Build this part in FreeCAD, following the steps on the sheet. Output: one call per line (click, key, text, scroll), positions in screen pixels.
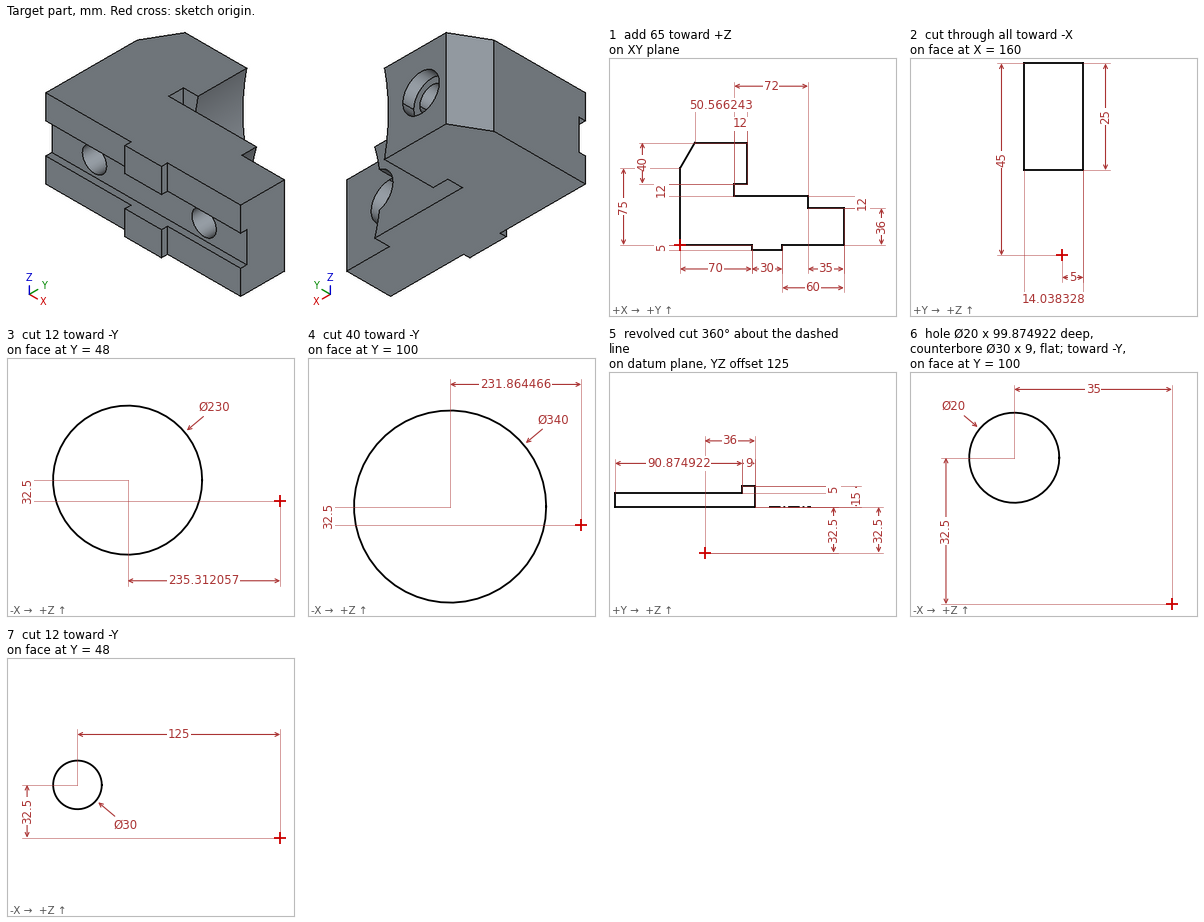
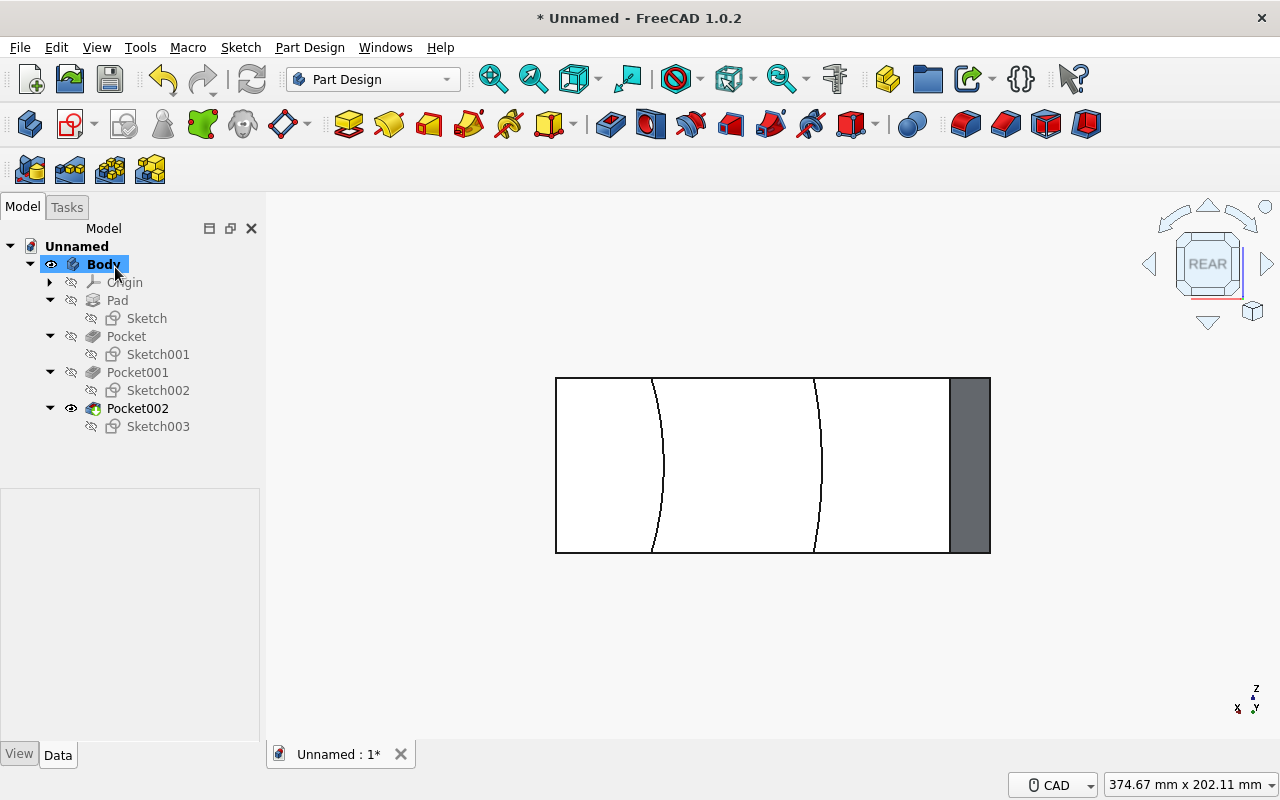
key(v)
key(f)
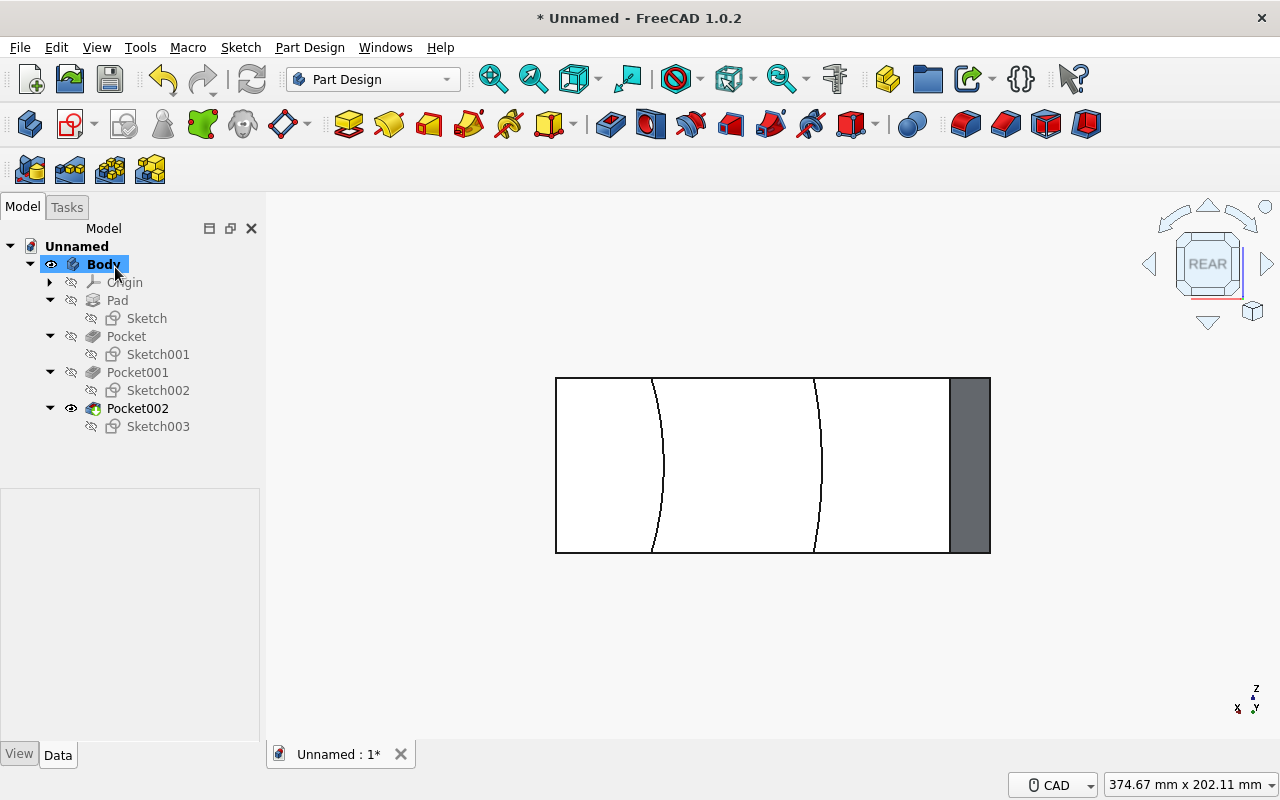
click(50, 282)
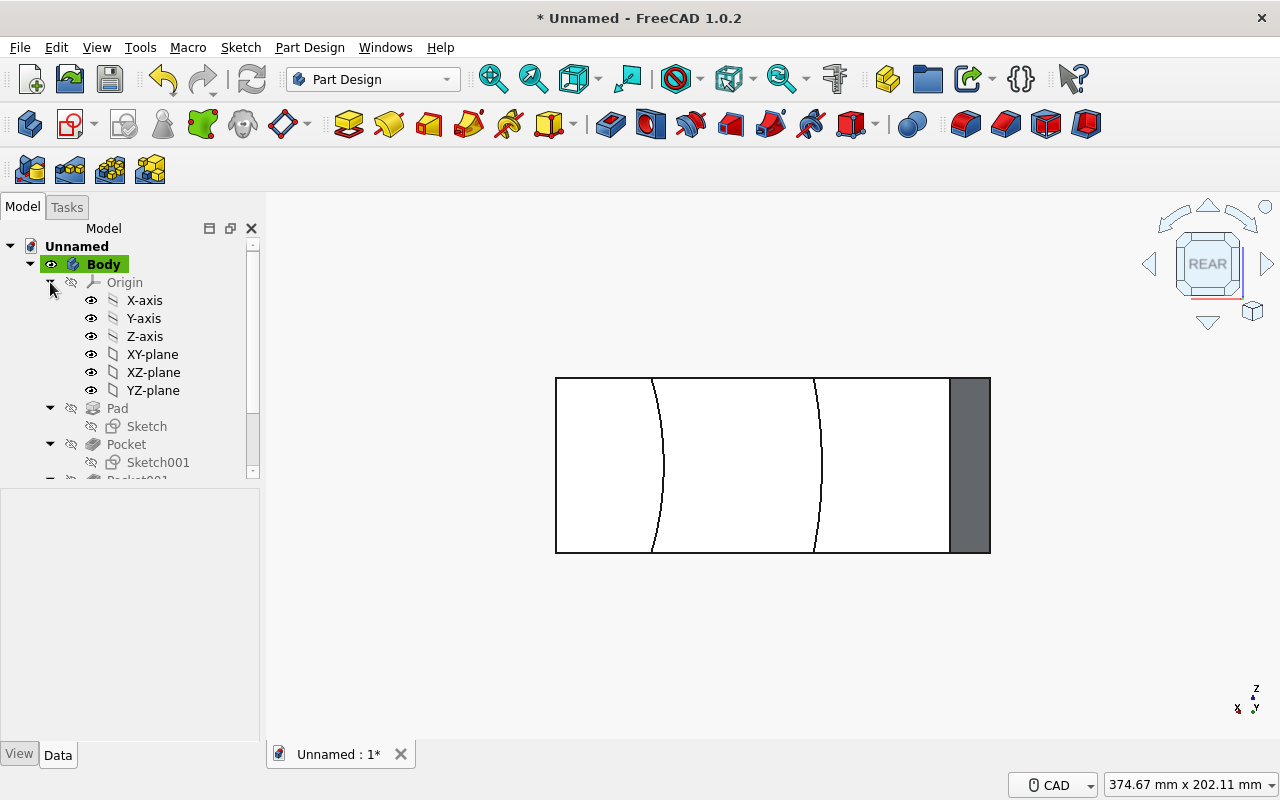
click(136, 390)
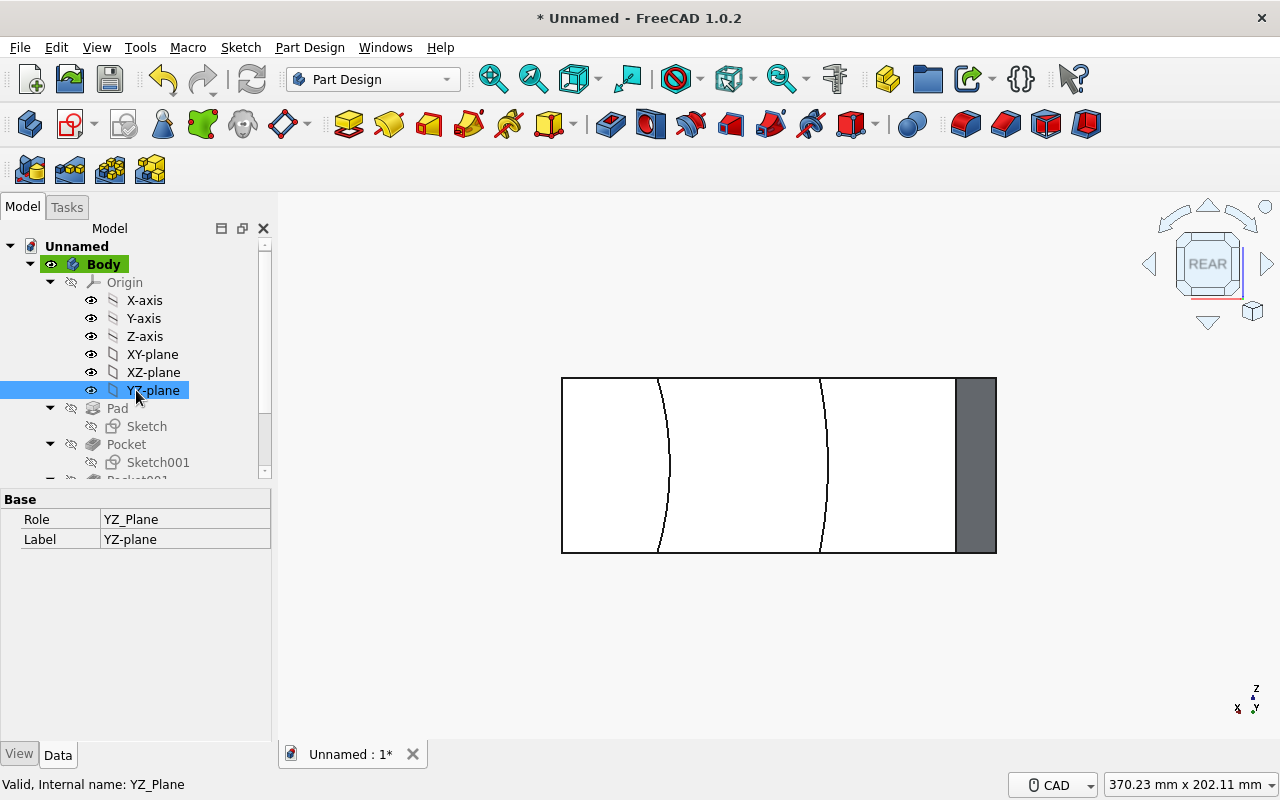
click(284, 124)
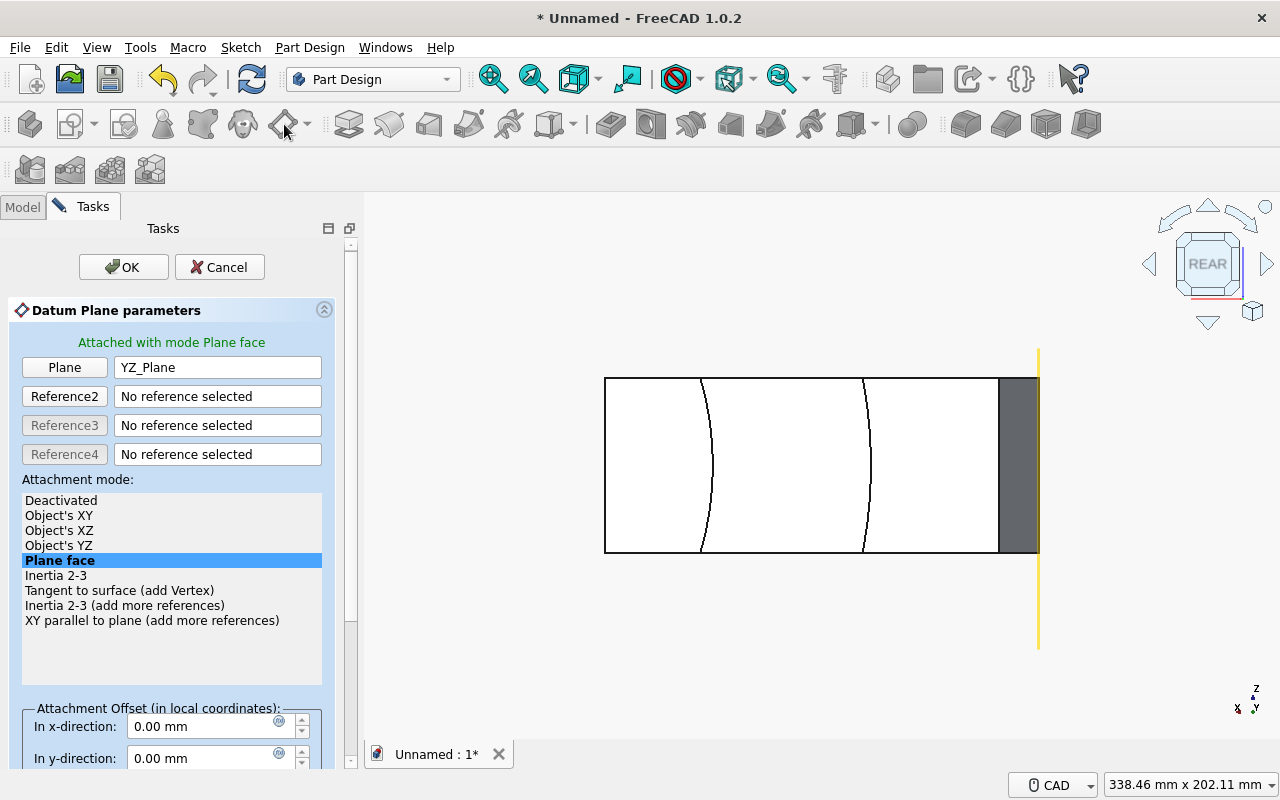
scroll(351, 503, down, 2)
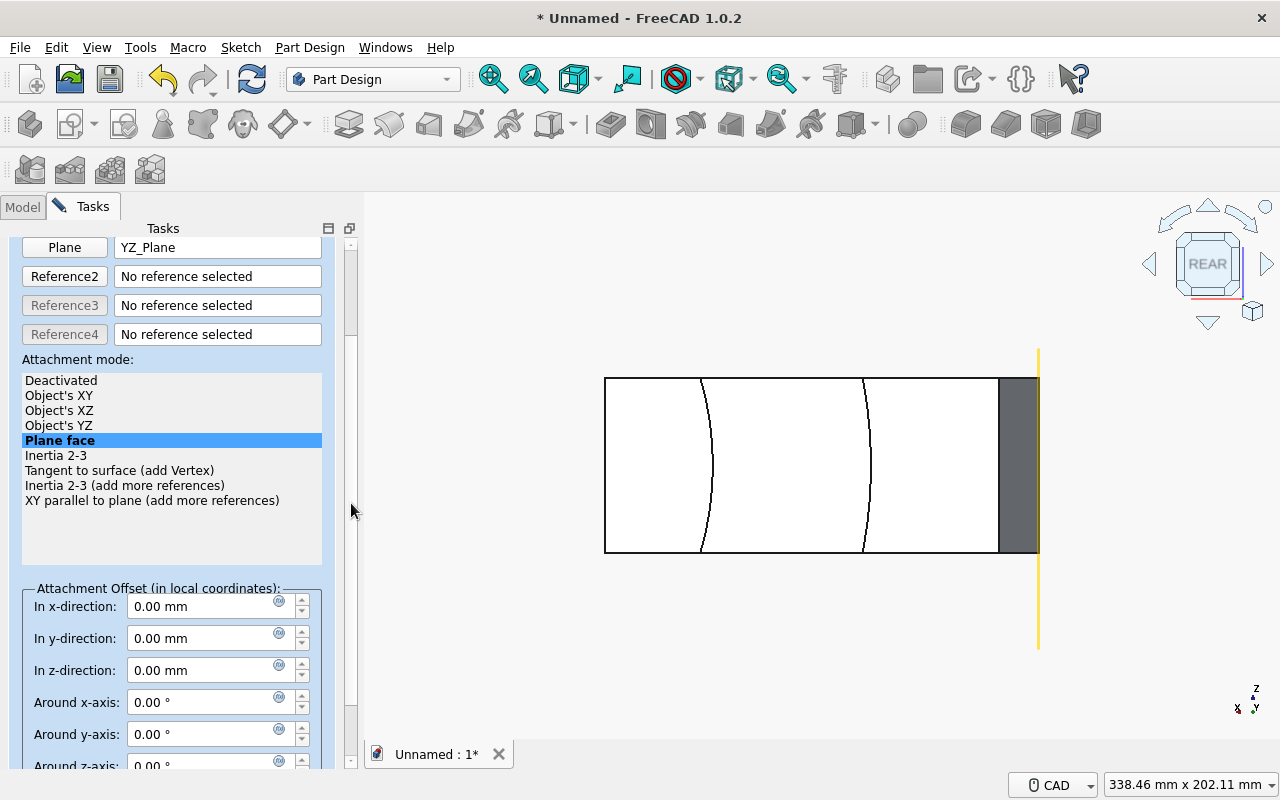
triple_click(210, 670)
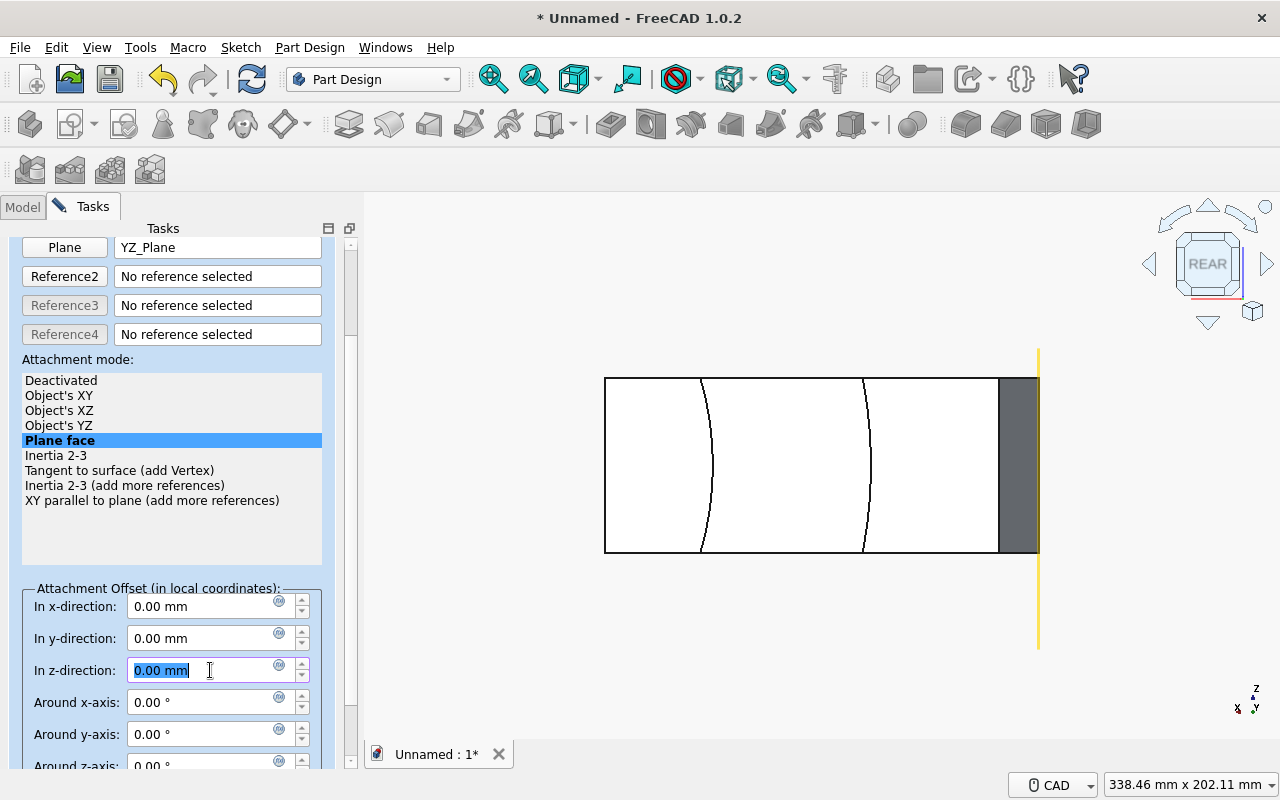
text(125)
key(Tab)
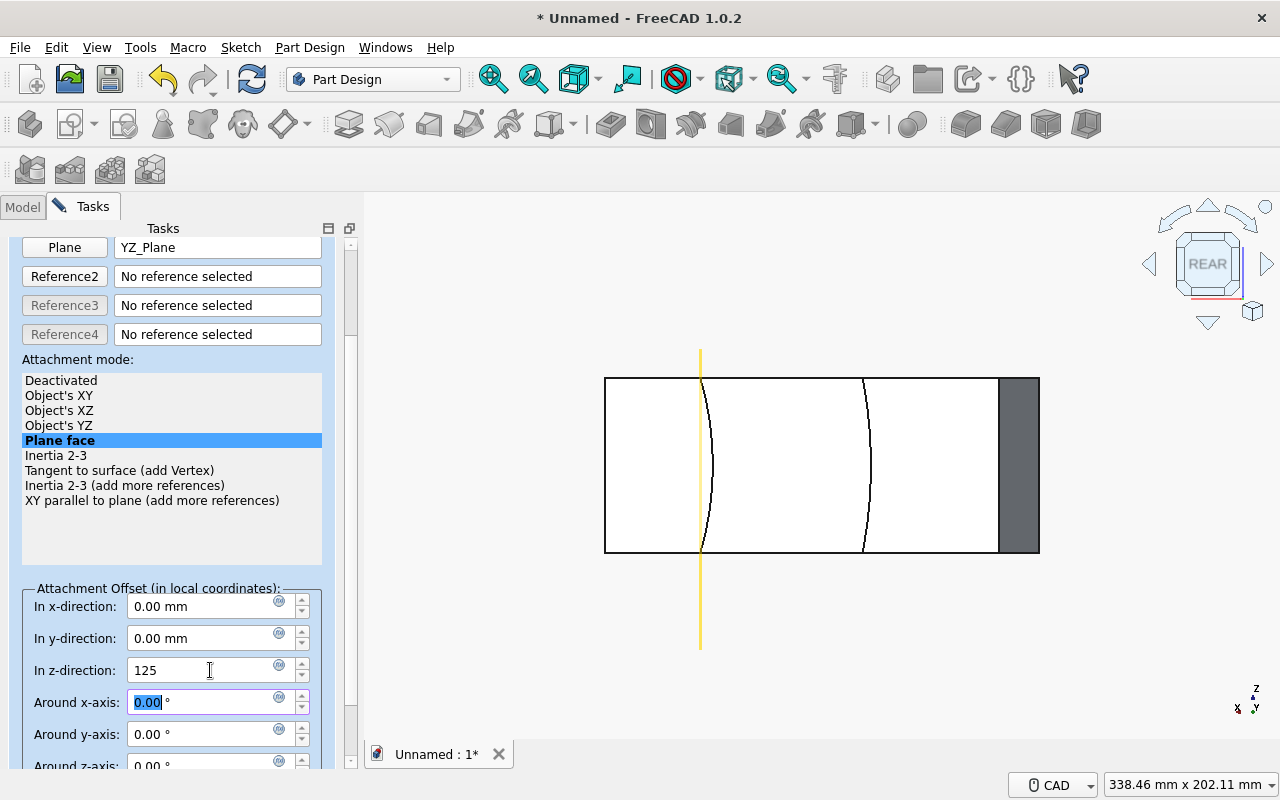
scroll(351, 503, up, 3)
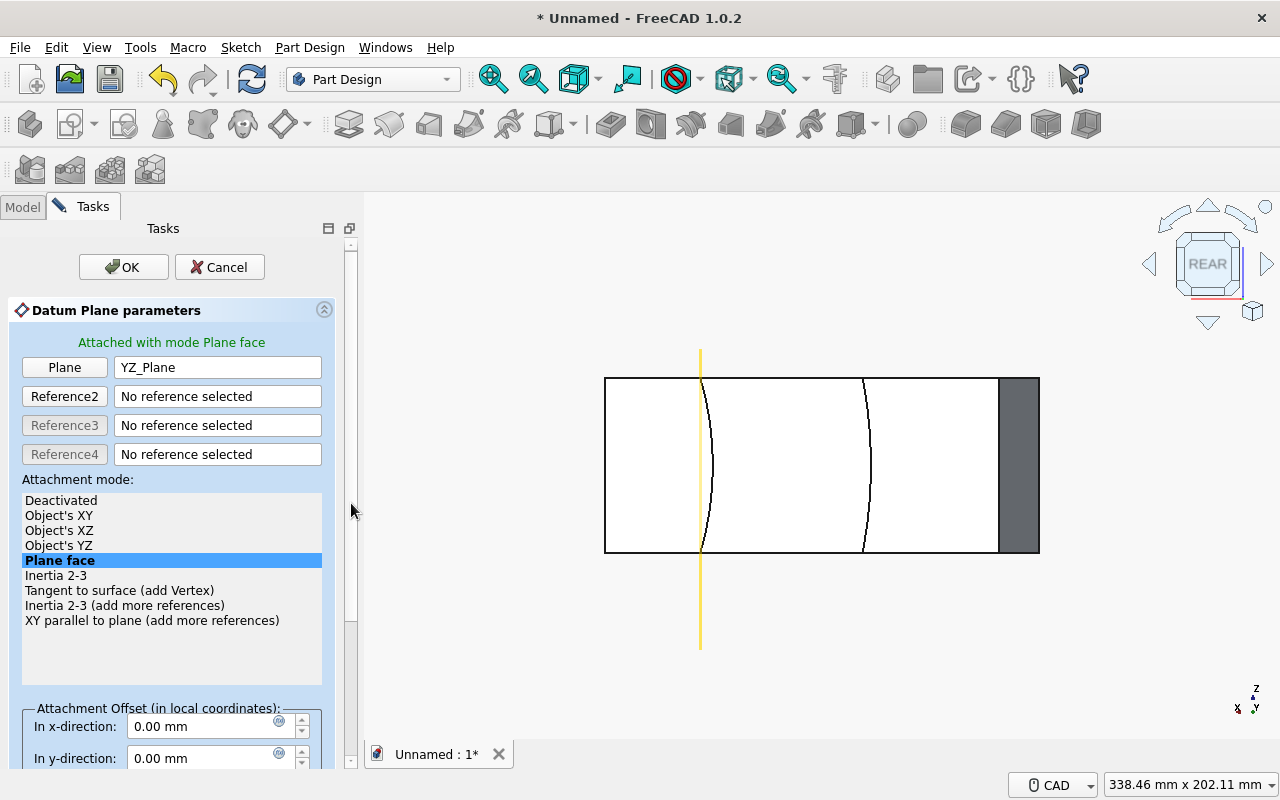
click(124, 267)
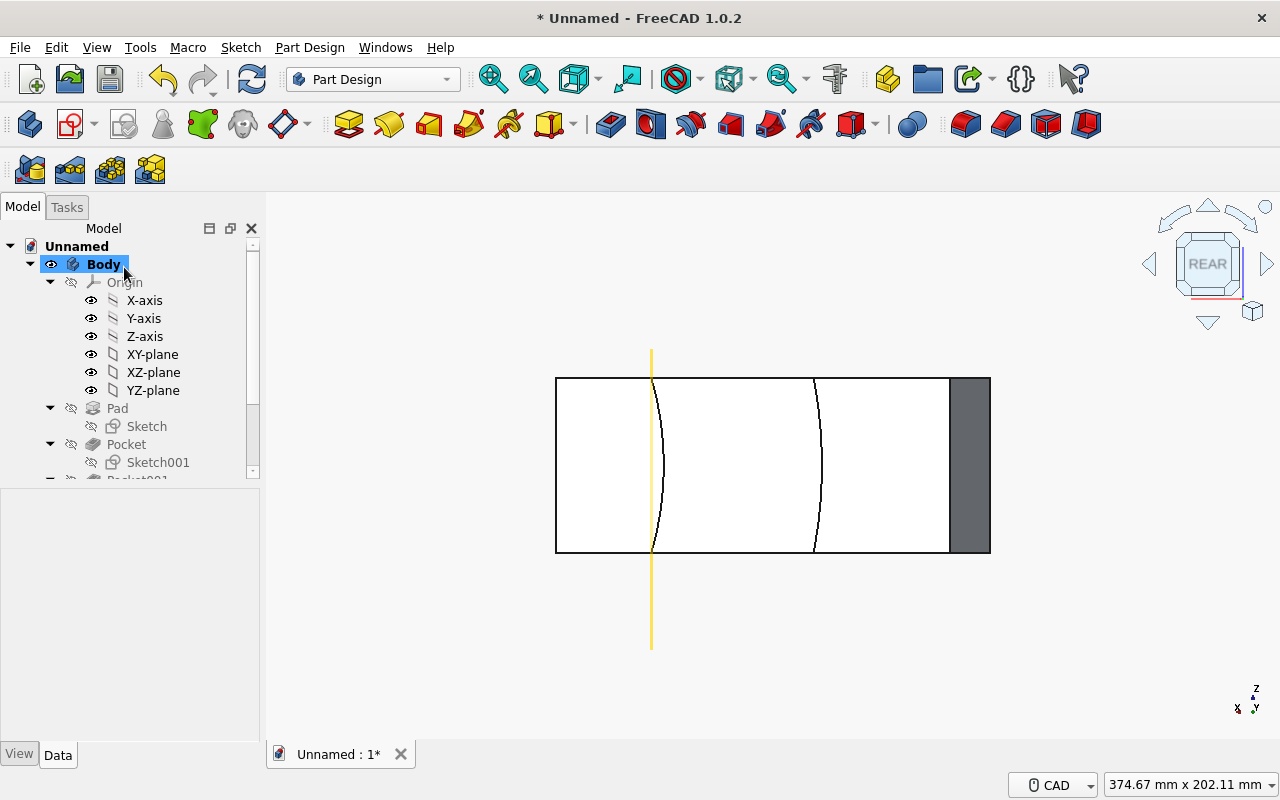
scroll(100, 350, down, 3)